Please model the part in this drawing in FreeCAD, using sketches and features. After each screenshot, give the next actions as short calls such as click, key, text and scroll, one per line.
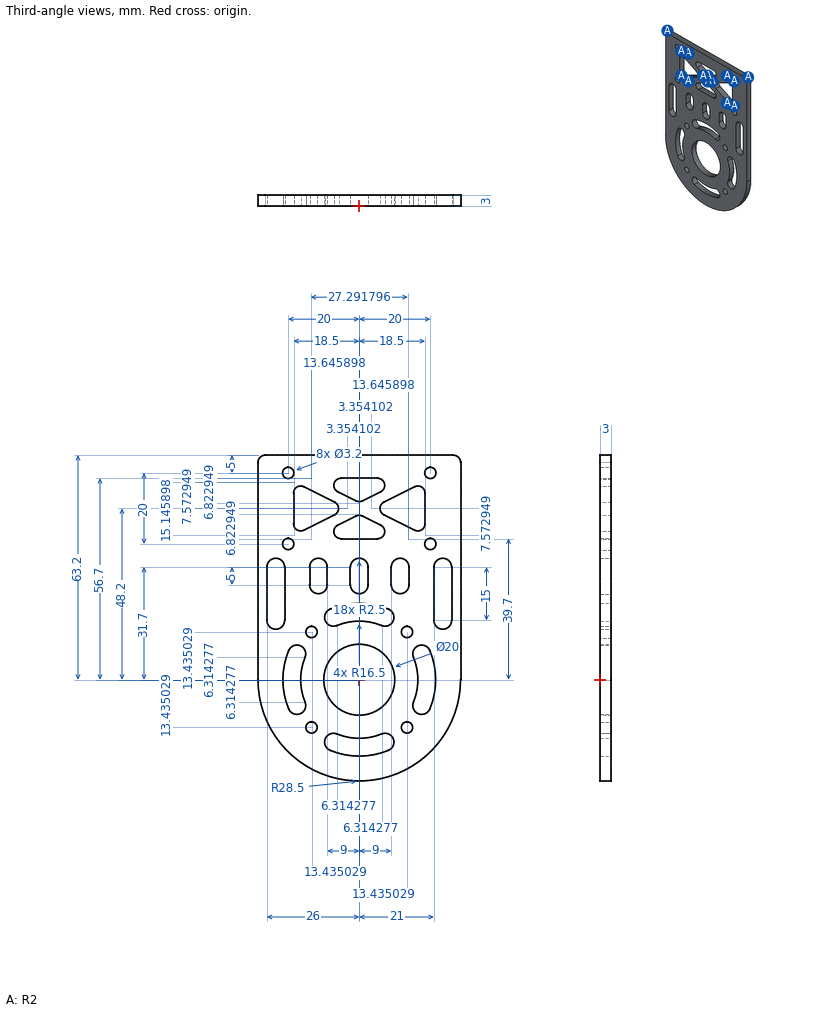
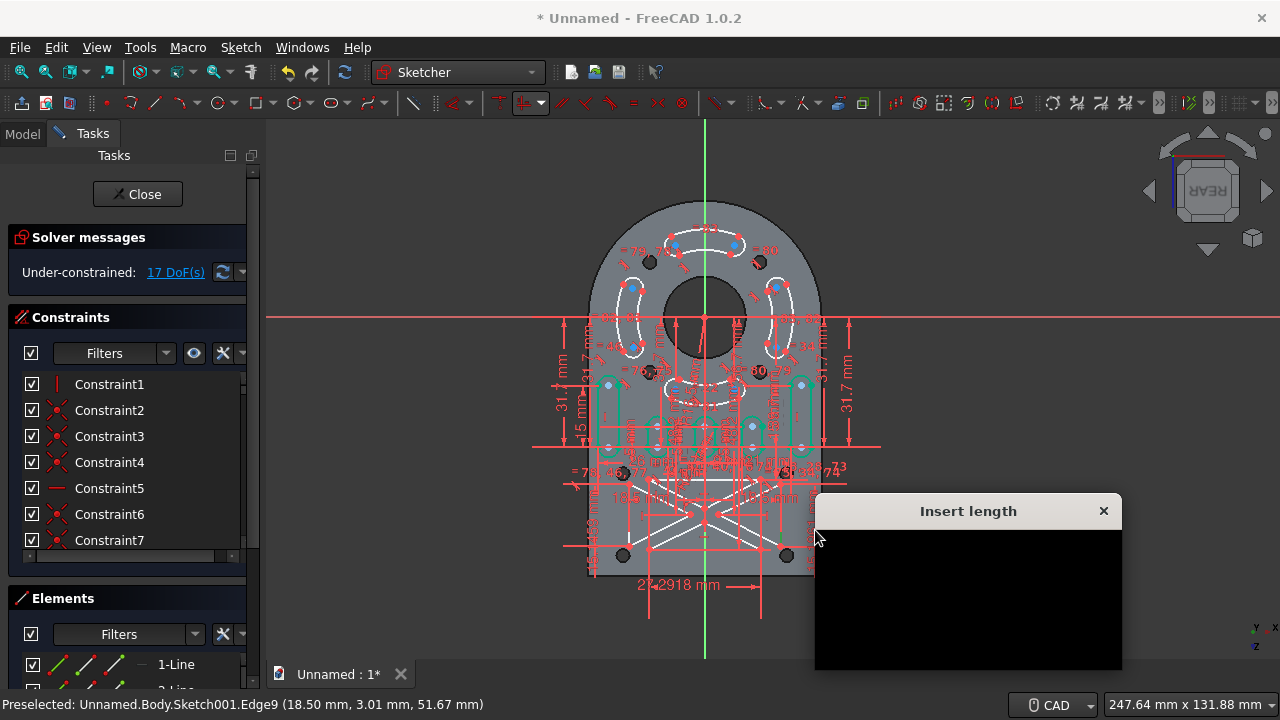
text(15.145898)
key(Return)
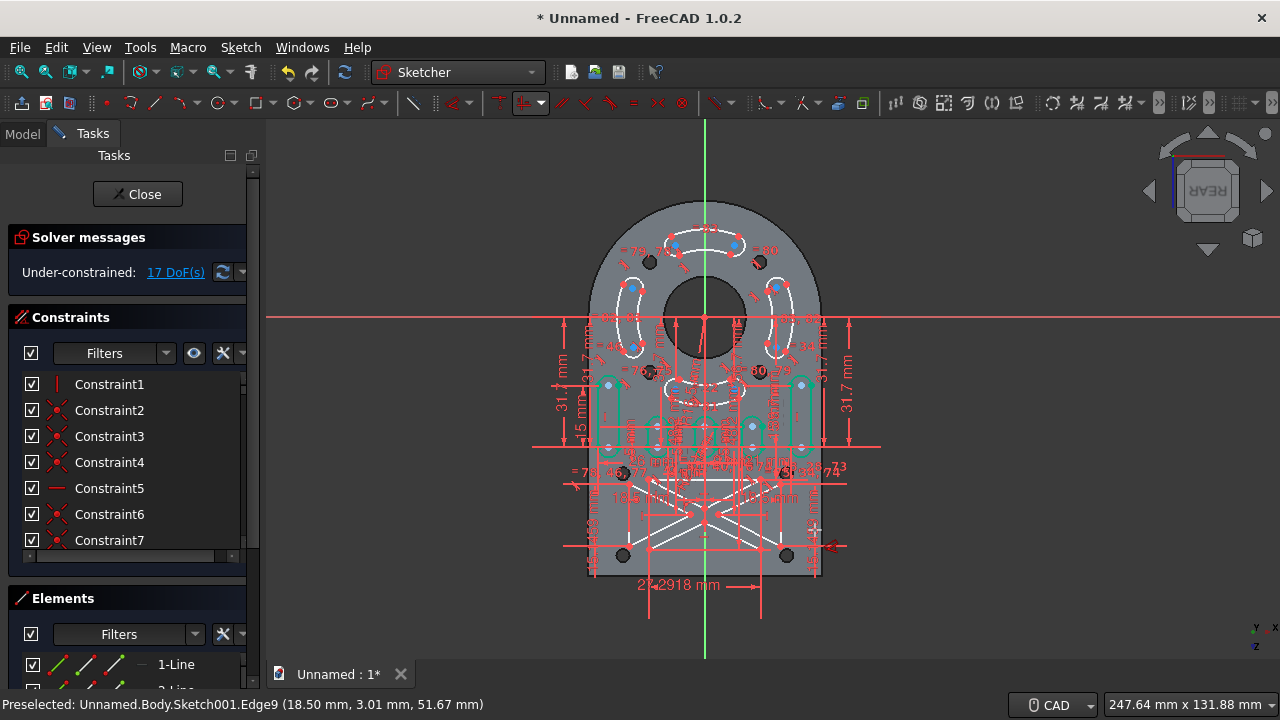
click(683, 550)
click(679, 608)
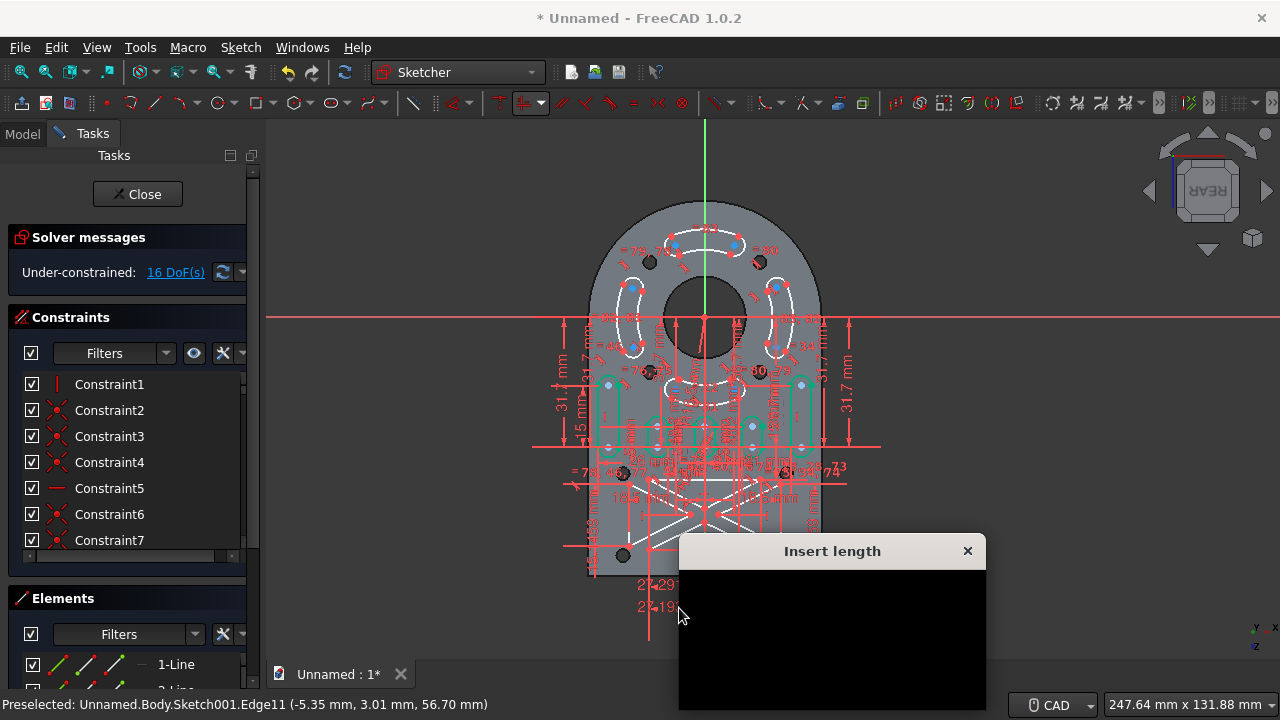
text(27.291796)
key(Return)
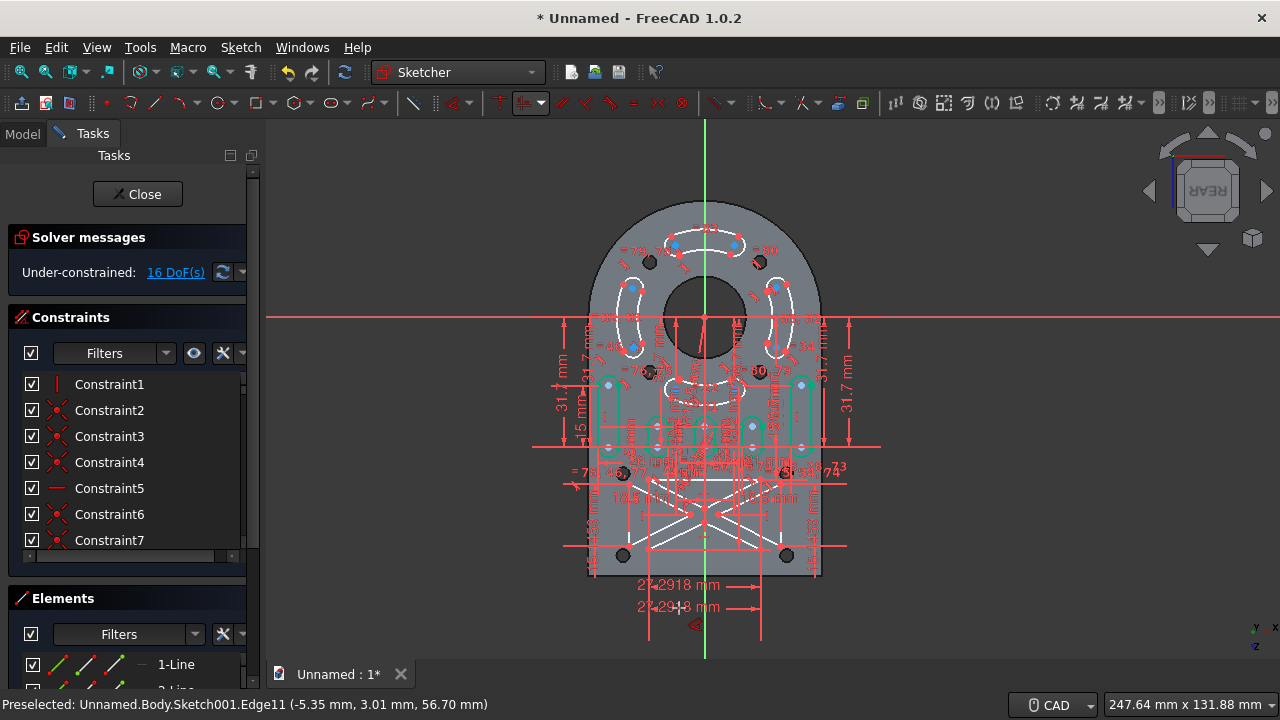
scroll(691, 515, up, 6)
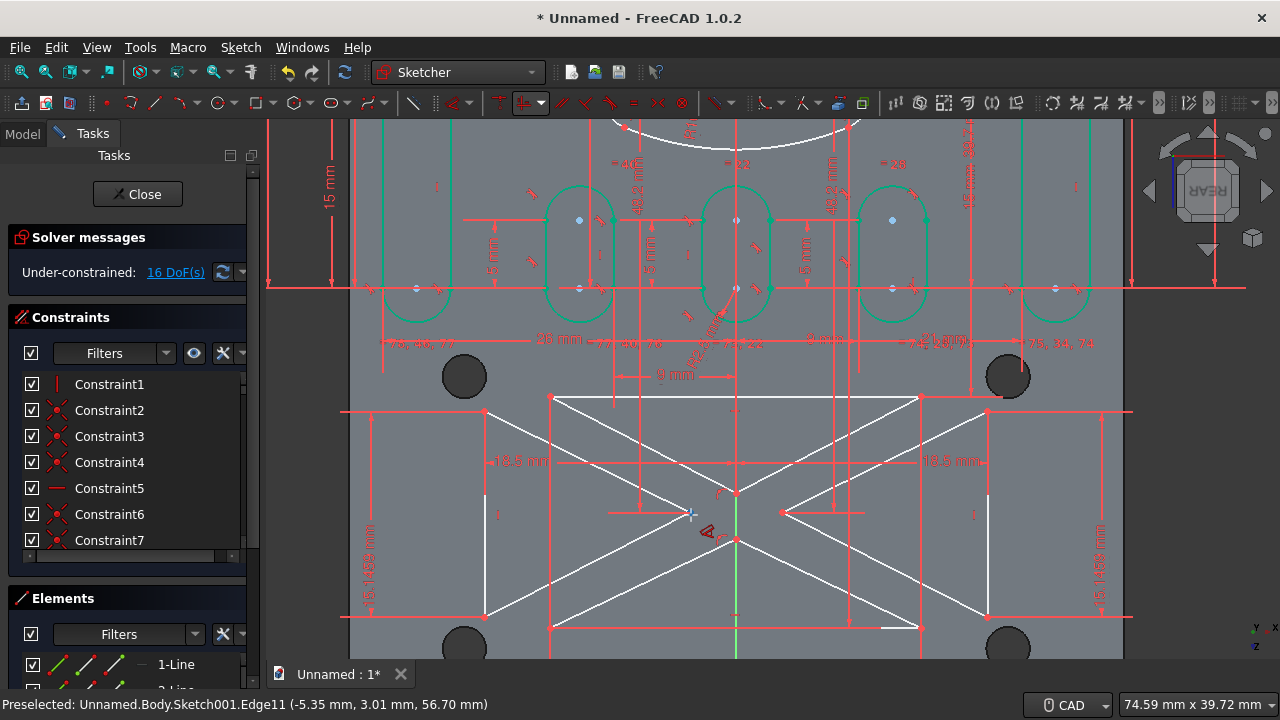
click(690, 513)
click(713, 571)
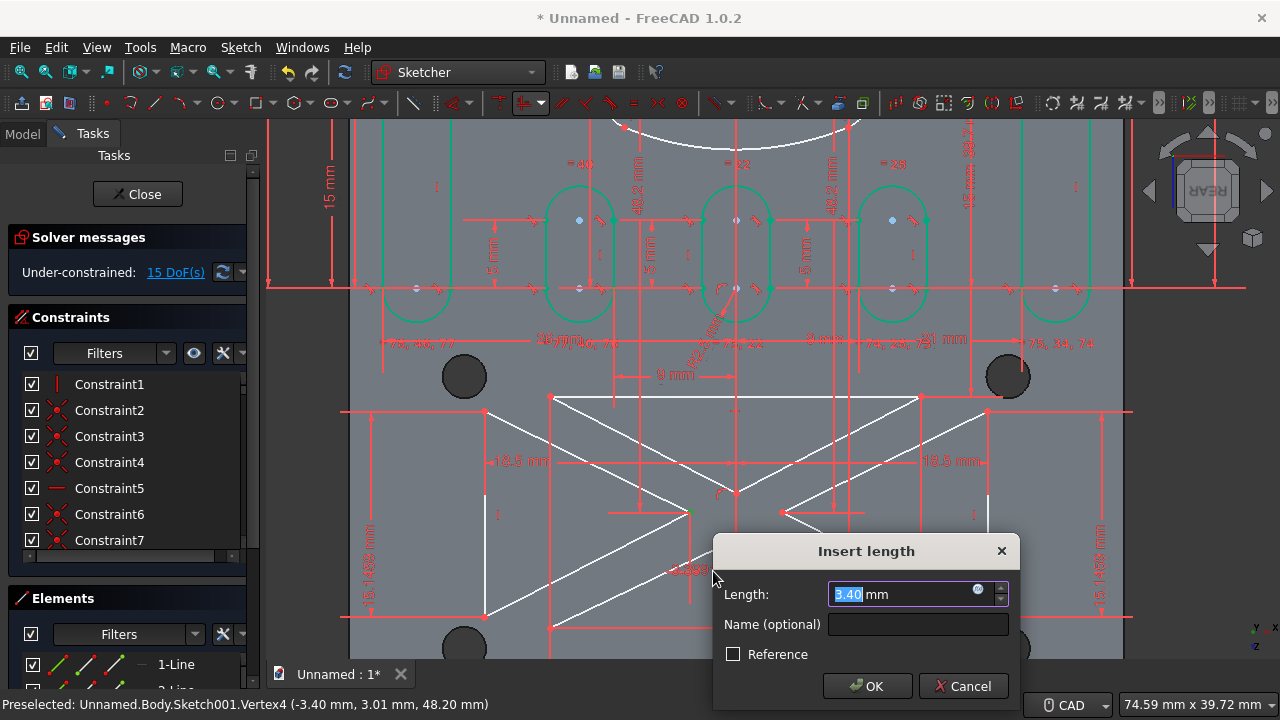
text(3.354102)
key(Return)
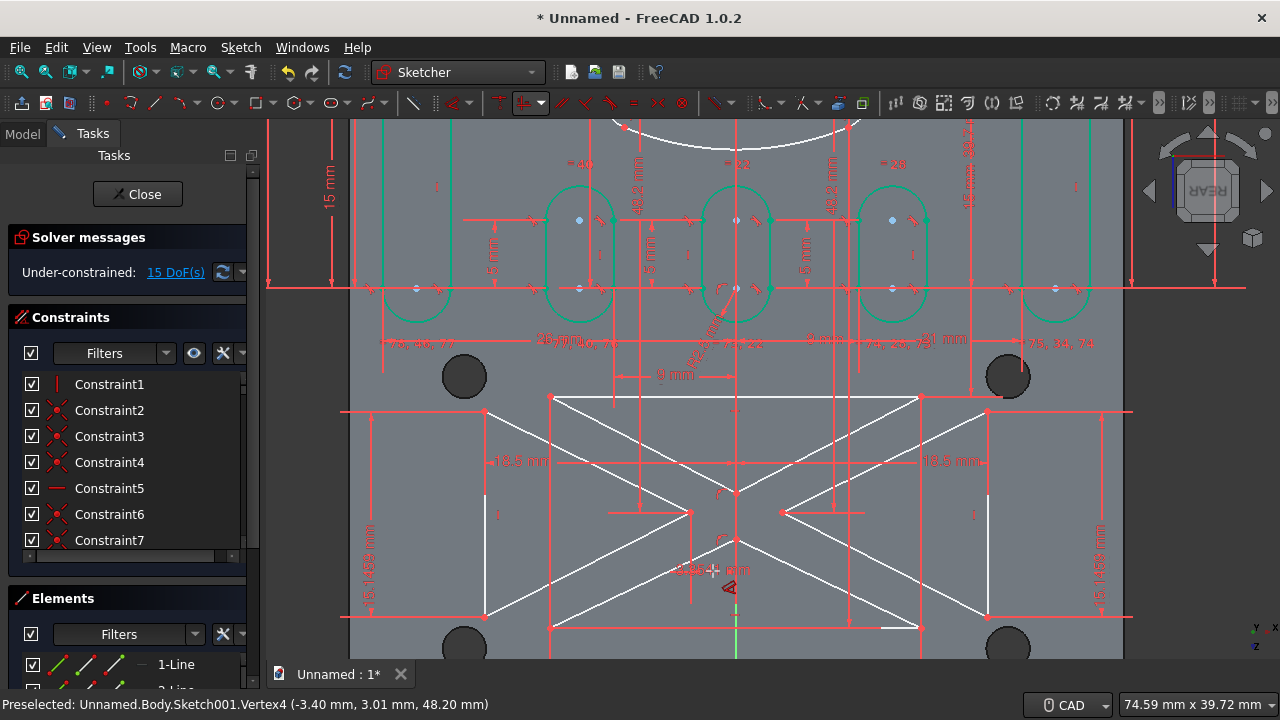
click(782, 513)
click(759, 595)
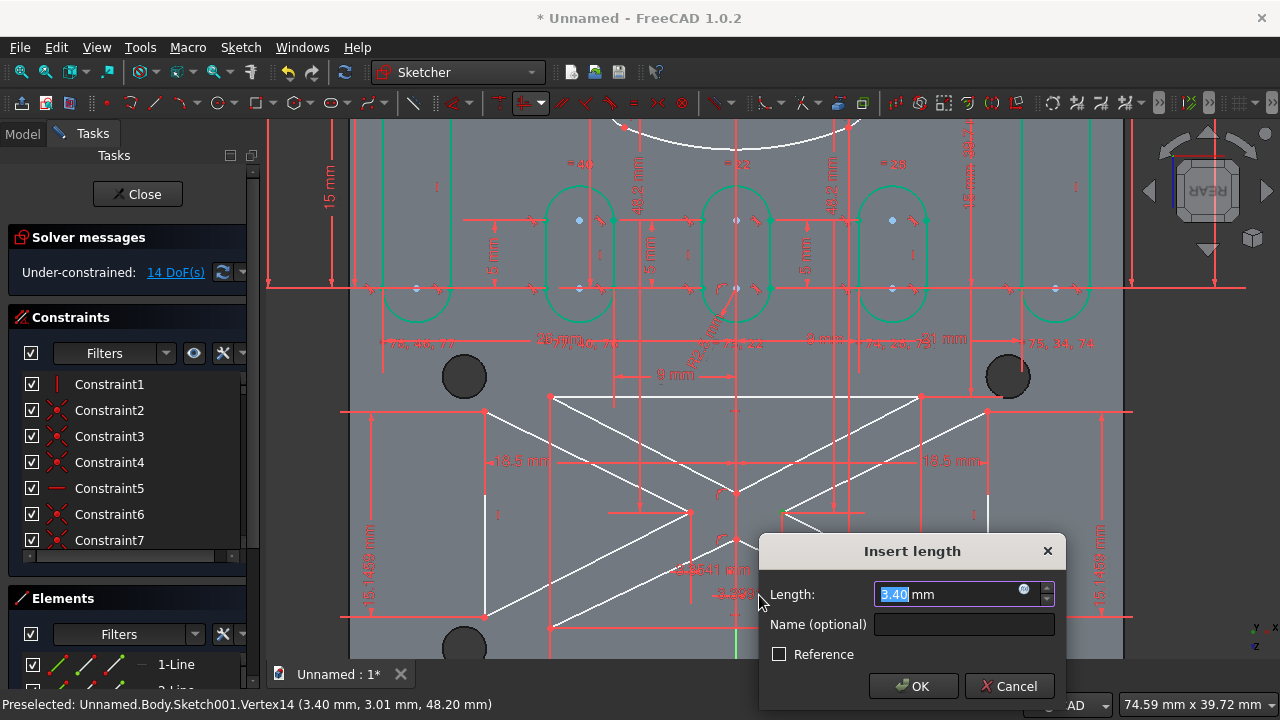
text(3.354102)
key(Return)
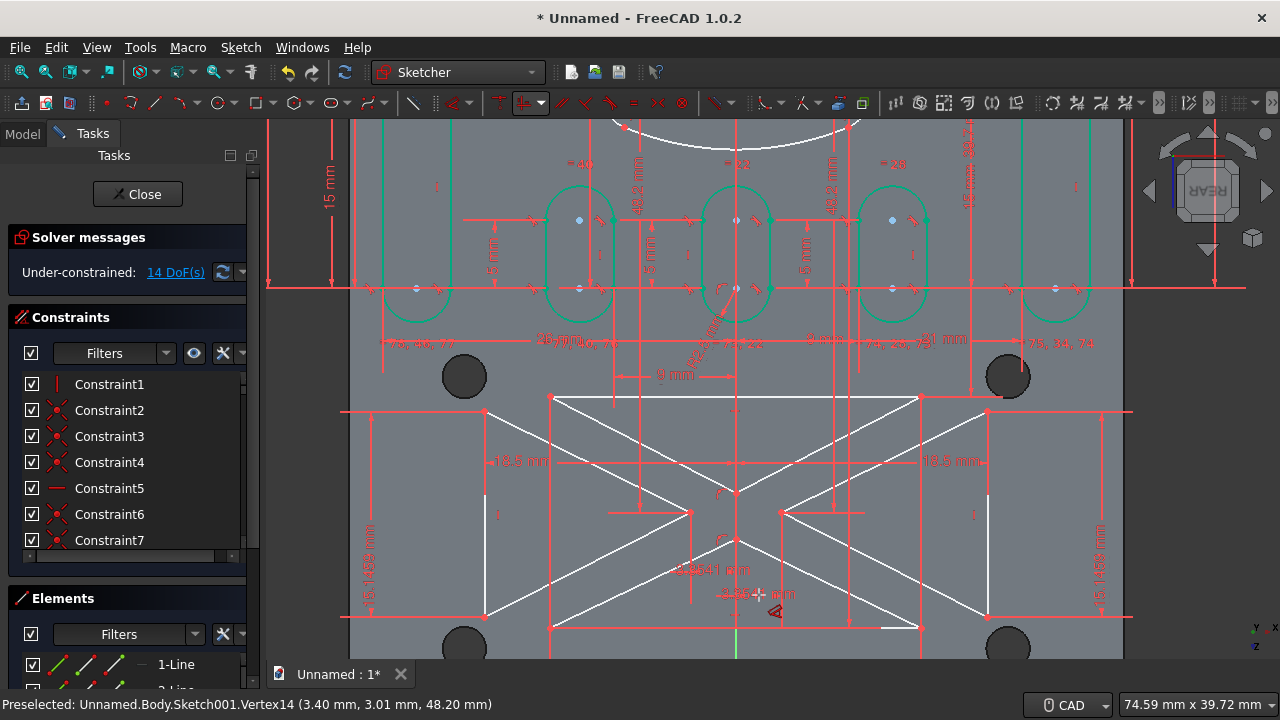
scroll(691, 515, down, 6)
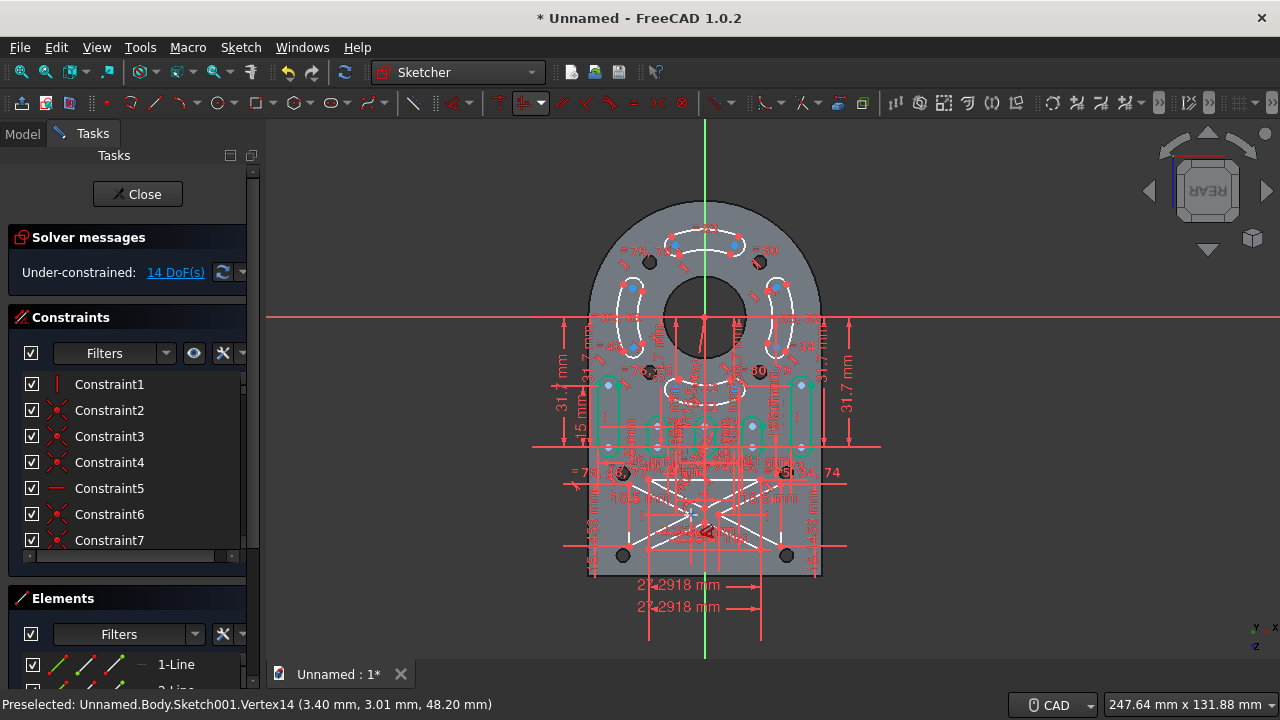
scroll(679, 380, up, 3)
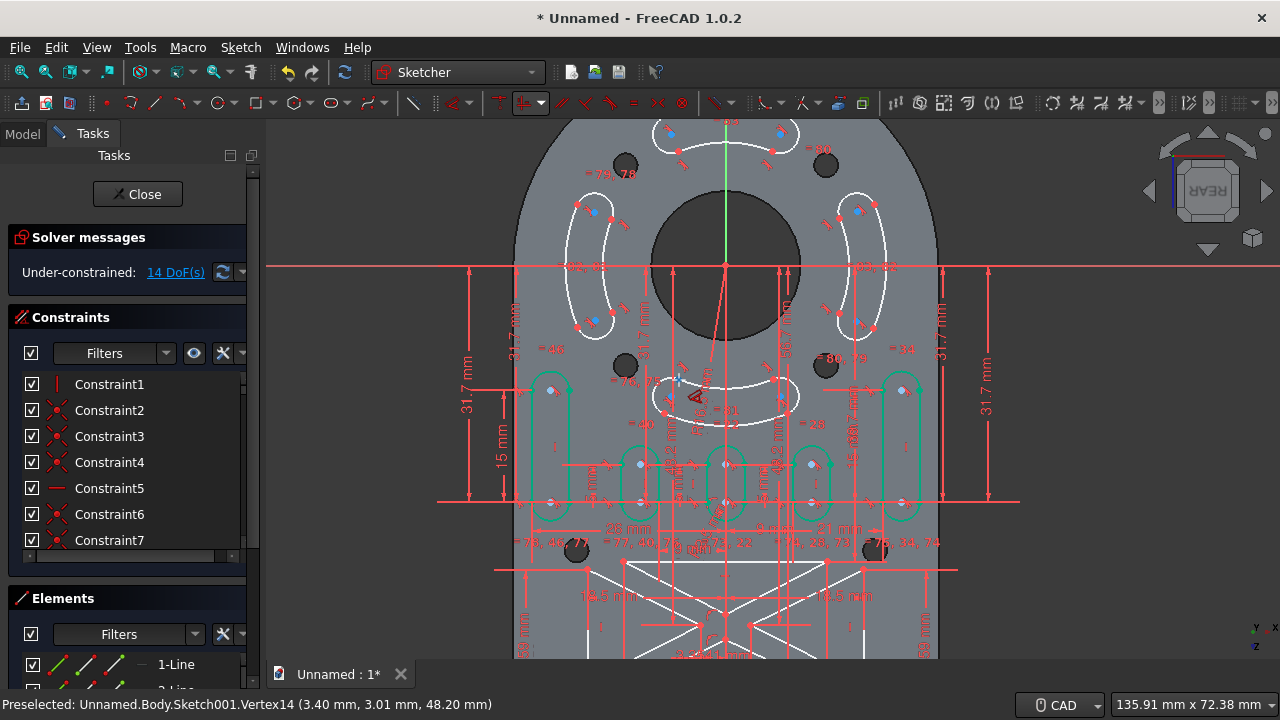
click(679, 379)
click(702, 232)